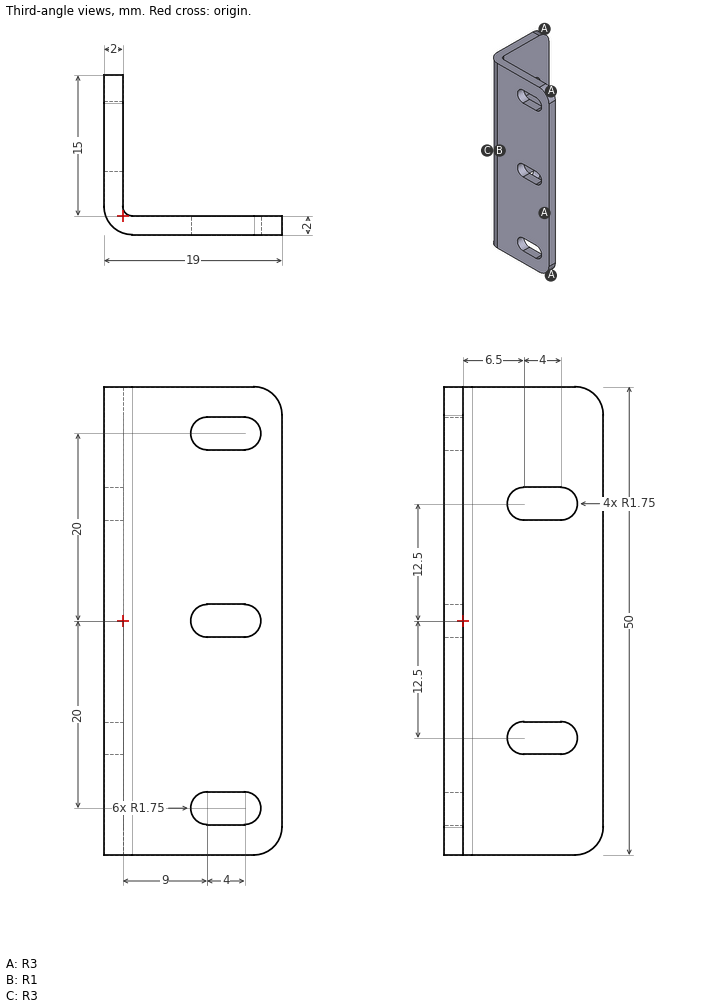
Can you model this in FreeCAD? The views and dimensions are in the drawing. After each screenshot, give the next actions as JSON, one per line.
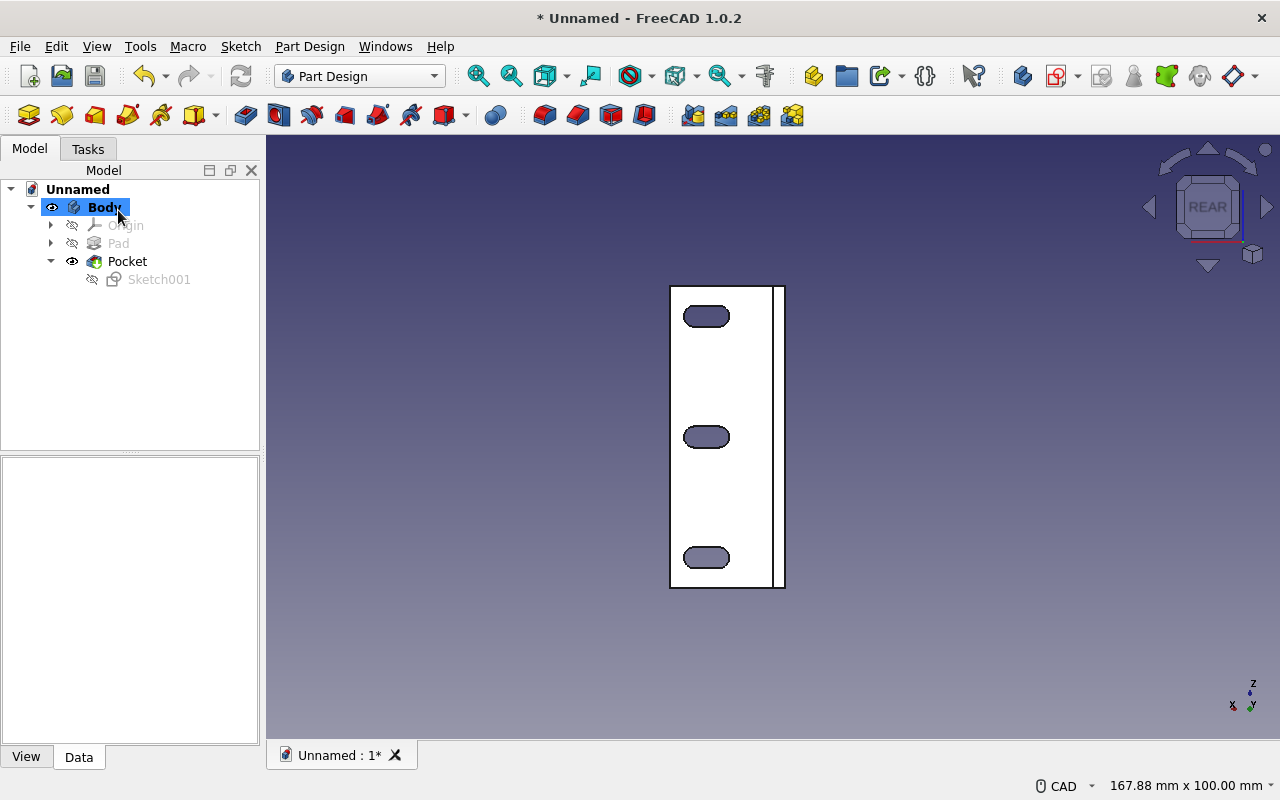
{"action": "left_click", "coordinate": [1056, 76]}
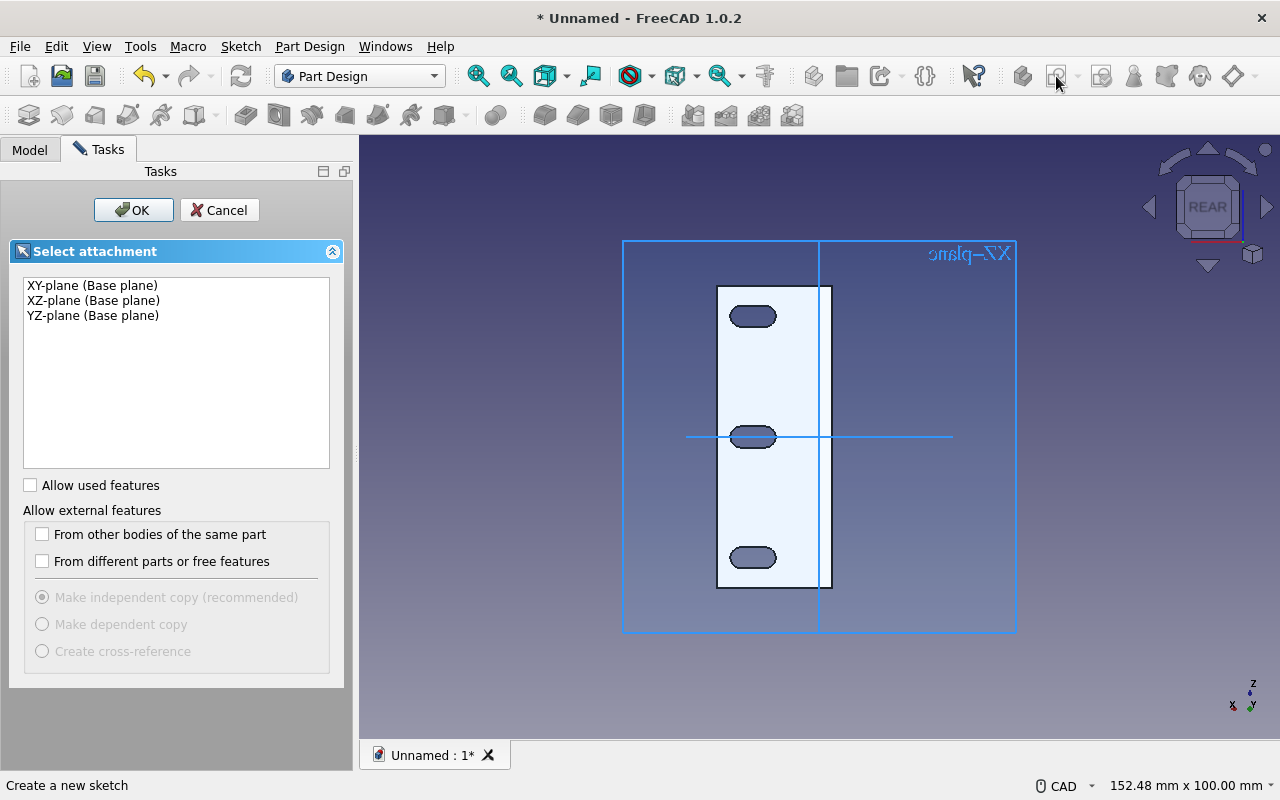
{"action": "left_click", "coordinate": [84, 316]}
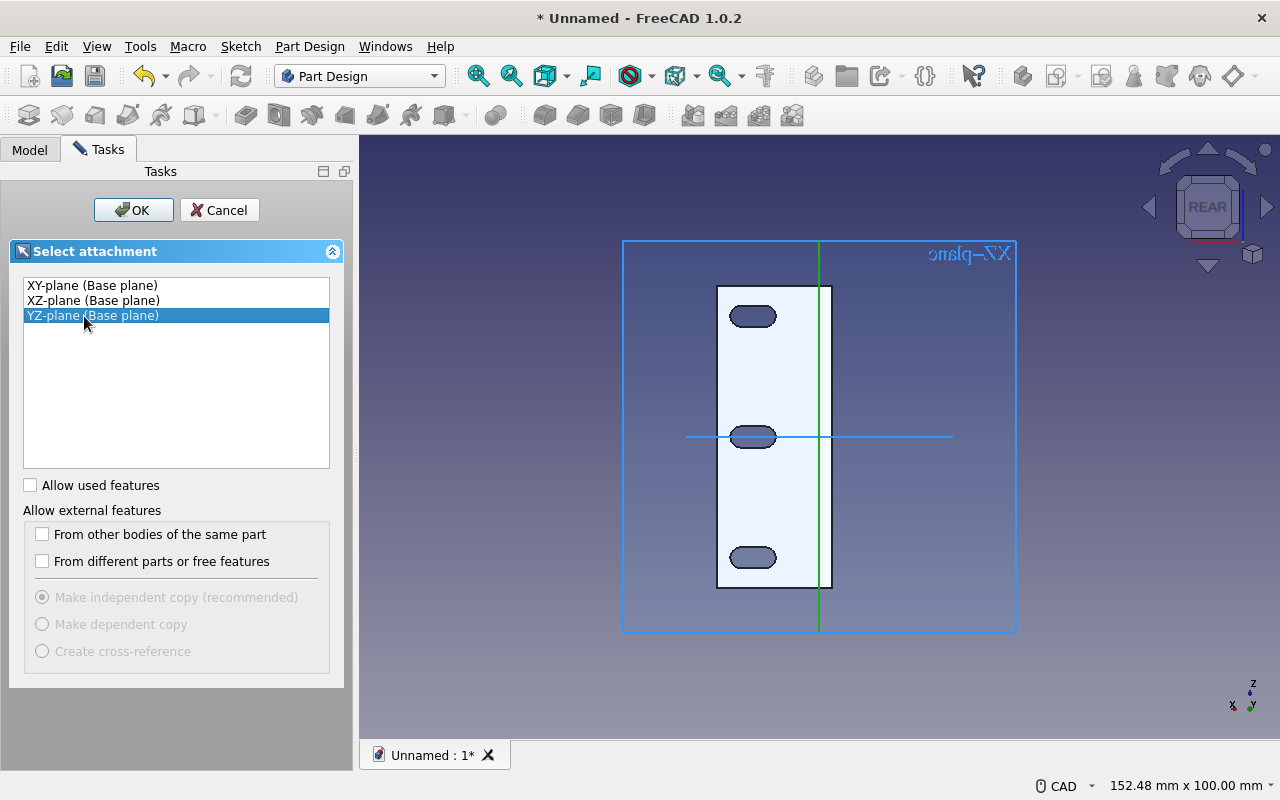
{"action": "left_click", "coordinate": [134, 210]}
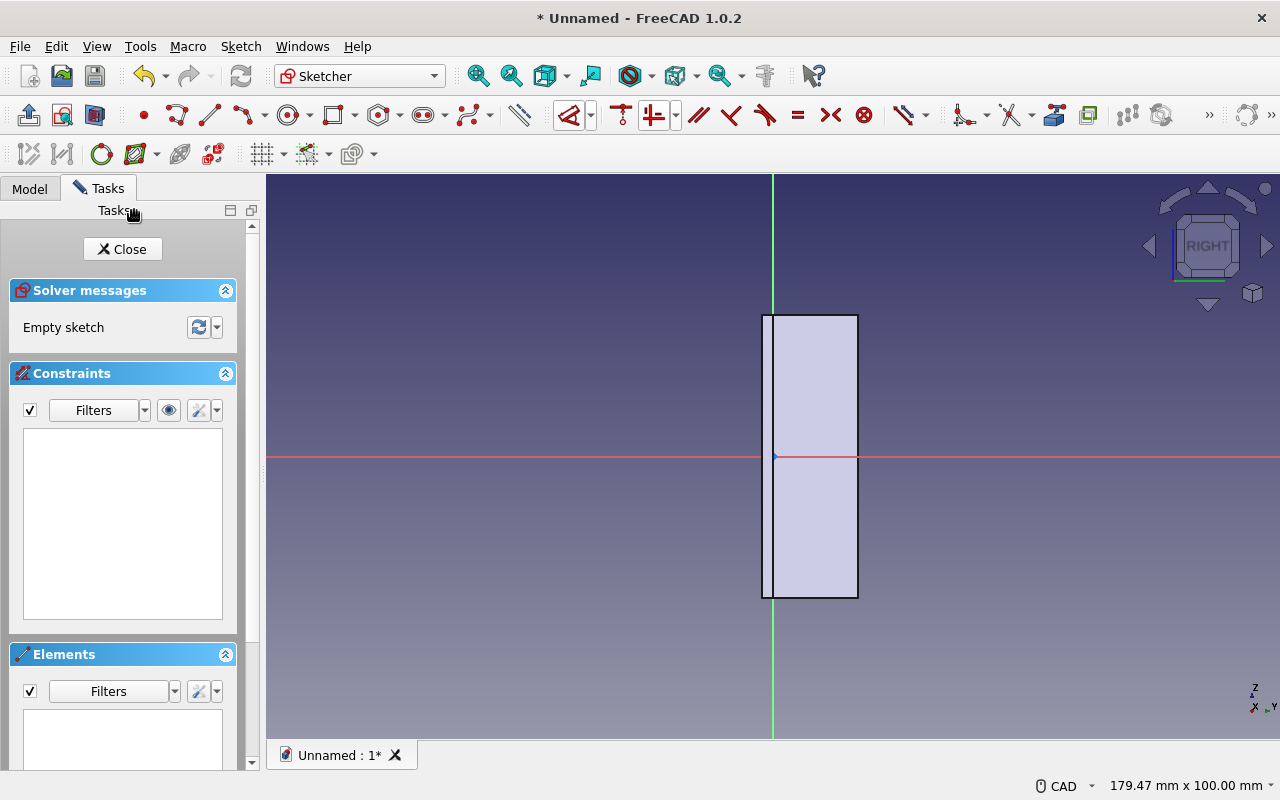
{"action": "left_click", "coordinate": [95, 116]}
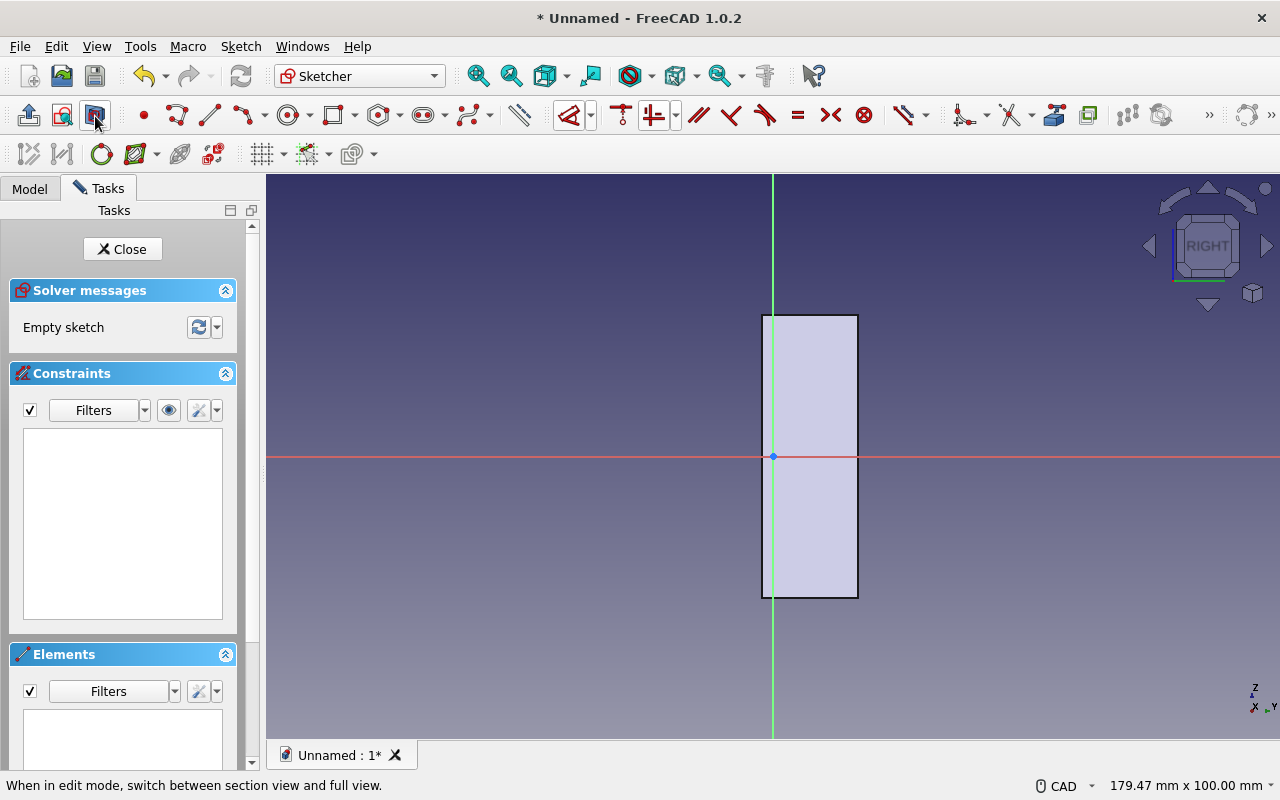
{"action": "scroll", "coordinate": [892, 457], "scroll_direction": "up", "scroll_amount": 4}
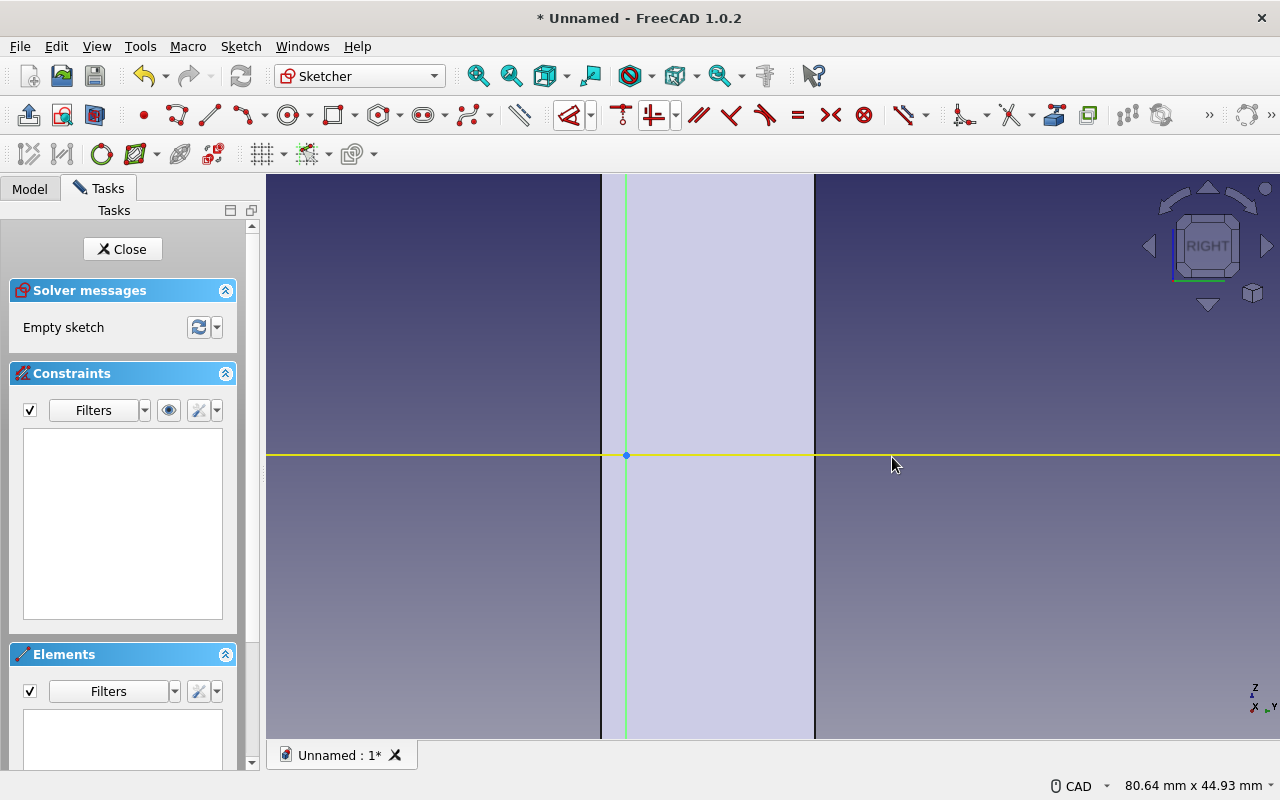
{"action": "left_click", "coordinate": [422, 116]}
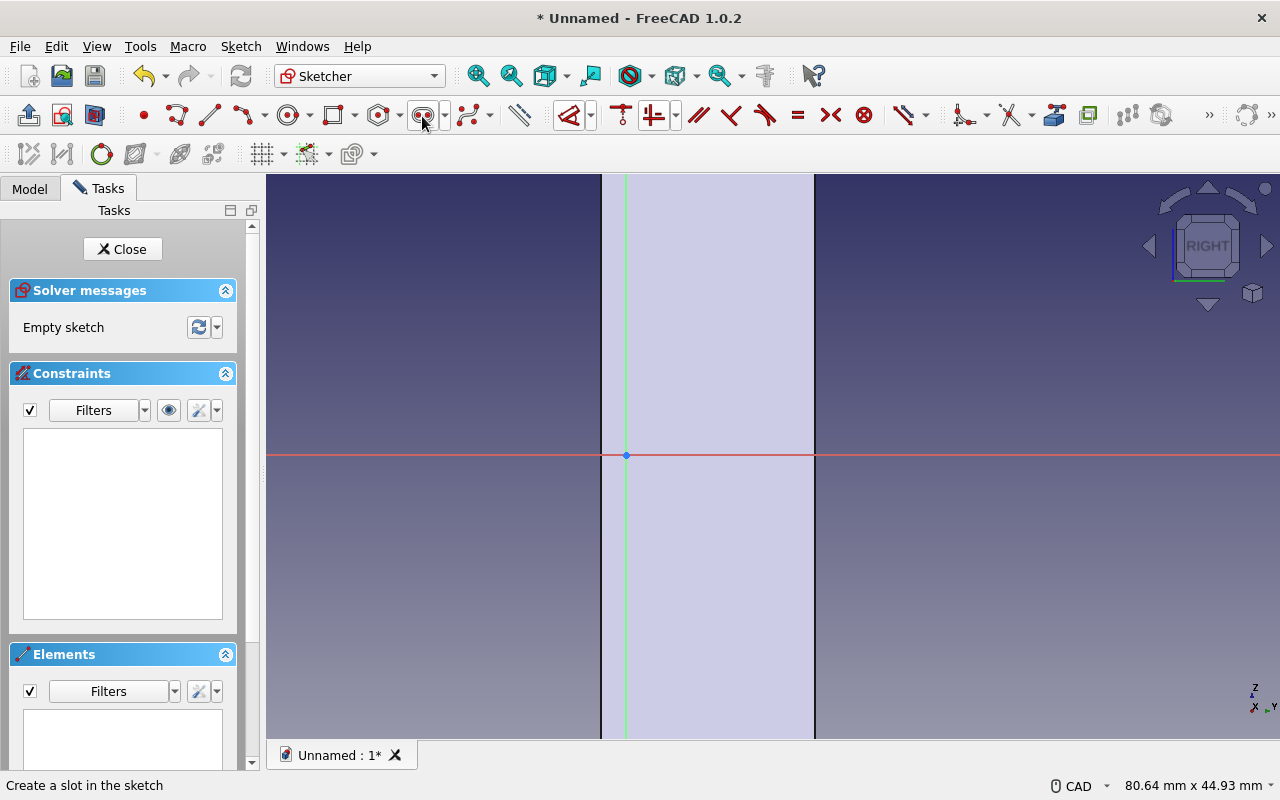
{"action": "left_click", "coordinate": [708, 298]}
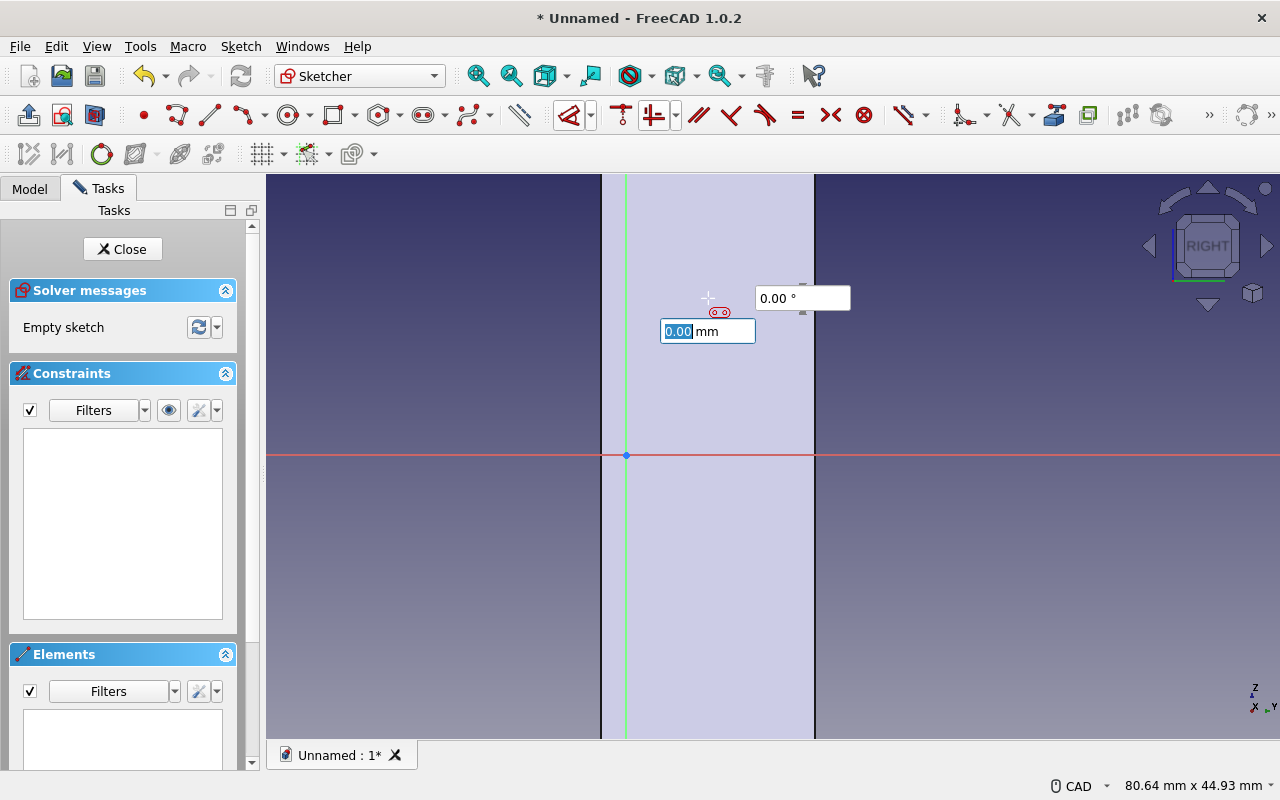
{"action": "left_click", "coordinate": [758, 298]}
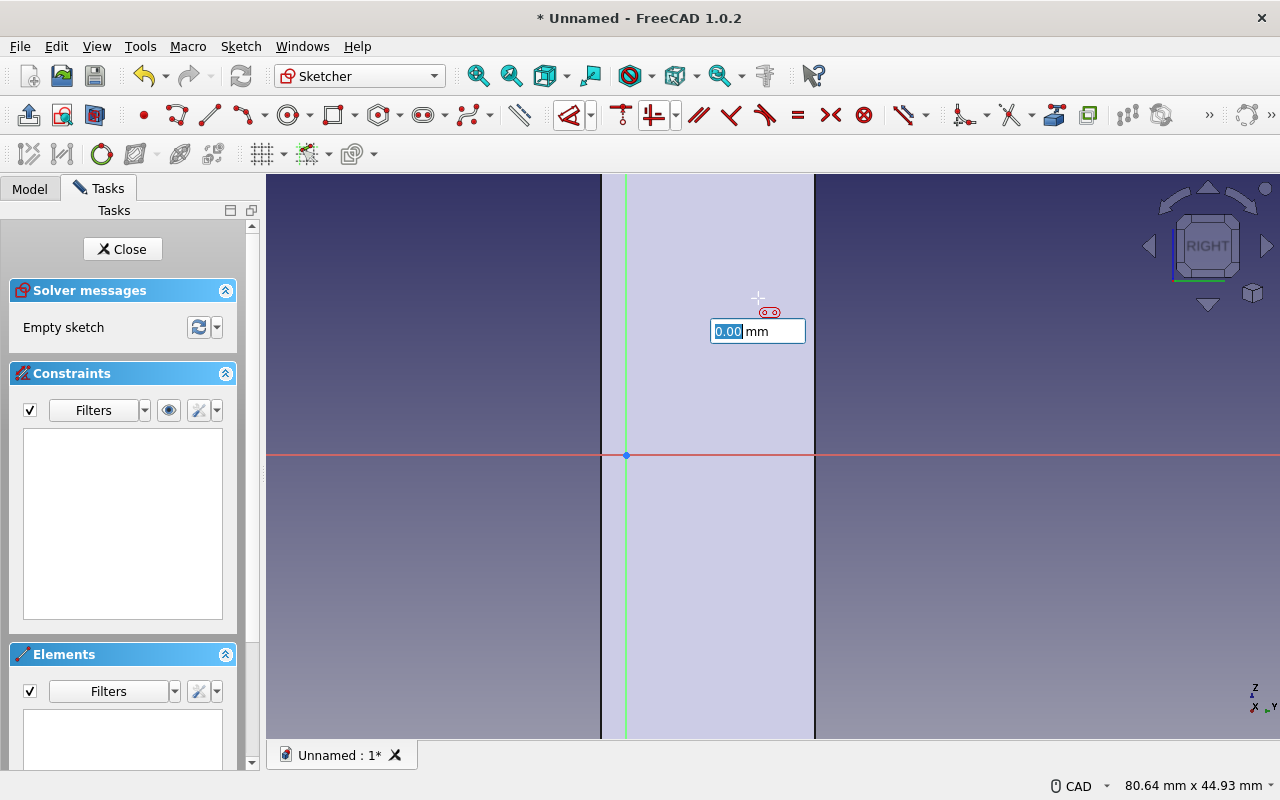
{"action": "left_click", "coordinate": [733, 320]}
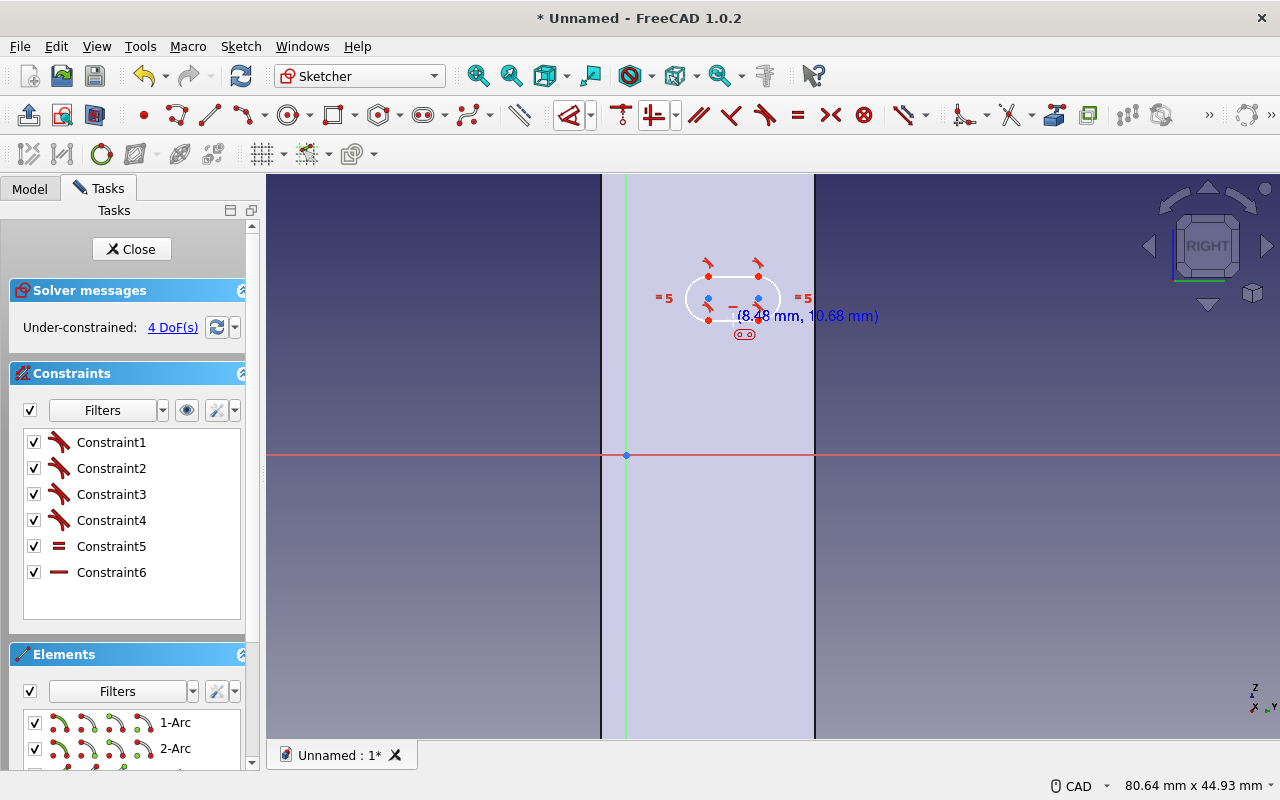
{"action": "left_click", "coordinate": [708, 612]}